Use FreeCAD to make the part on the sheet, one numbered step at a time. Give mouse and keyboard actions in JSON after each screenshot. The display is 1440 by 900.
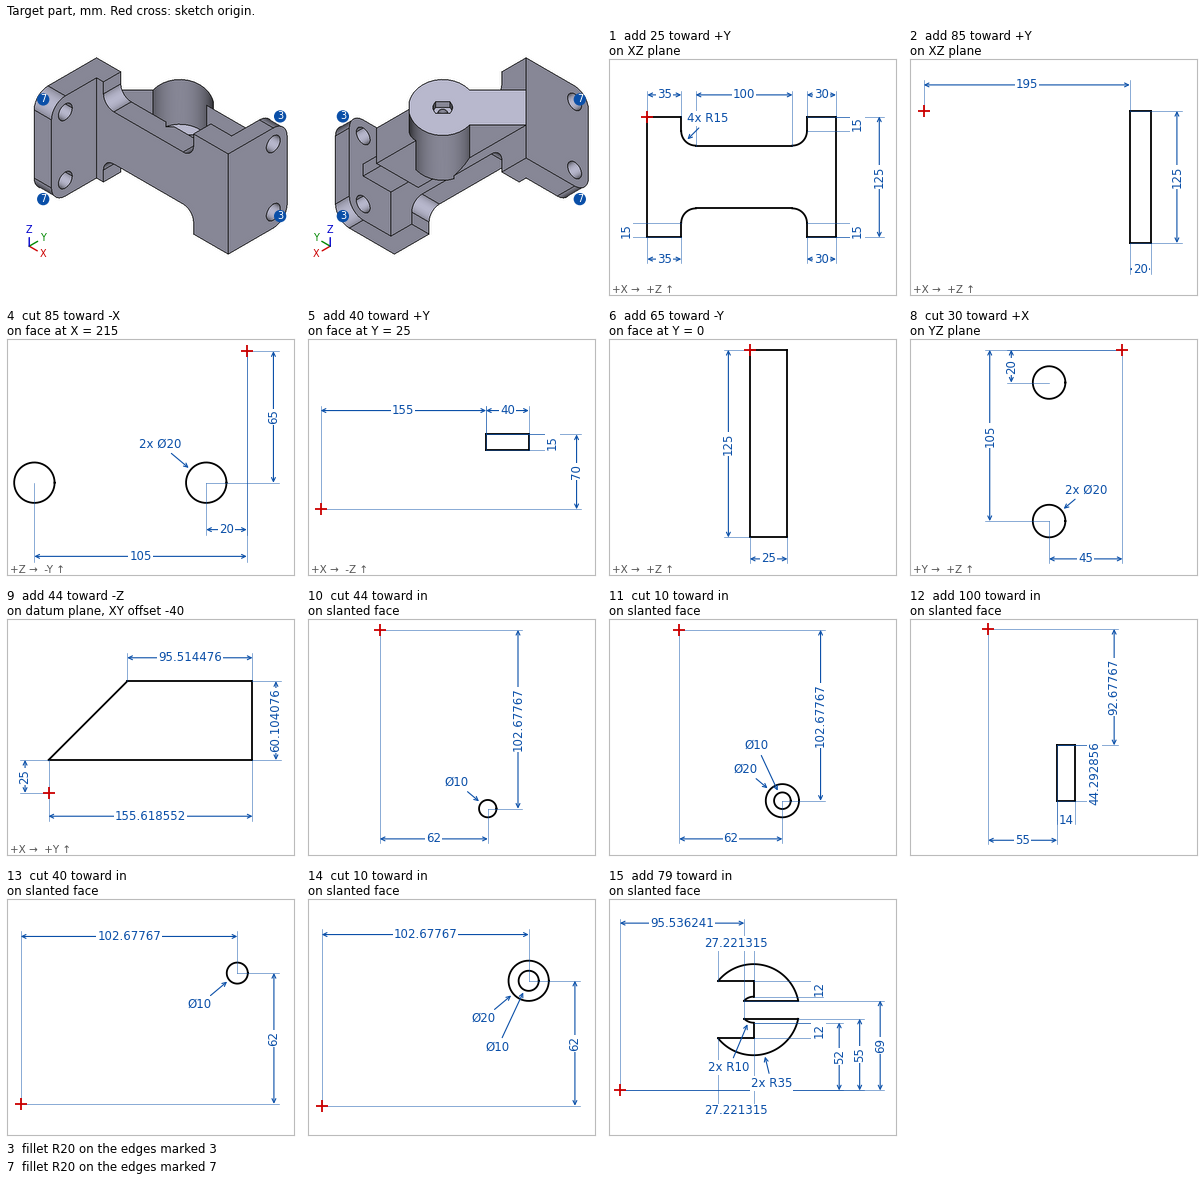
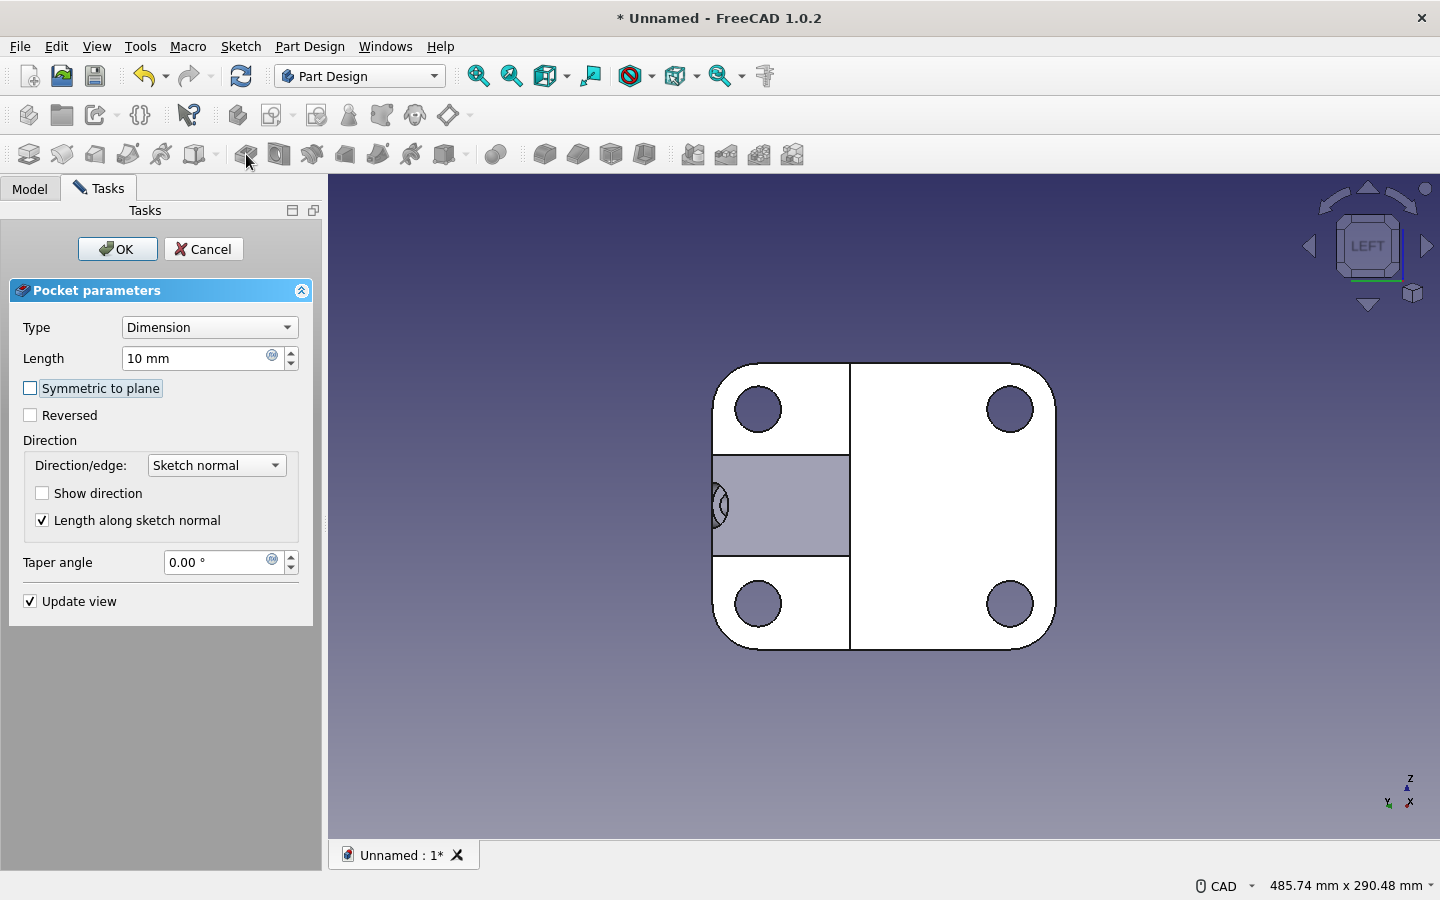
{"action": "left_click", "coordinate": [118, 249]}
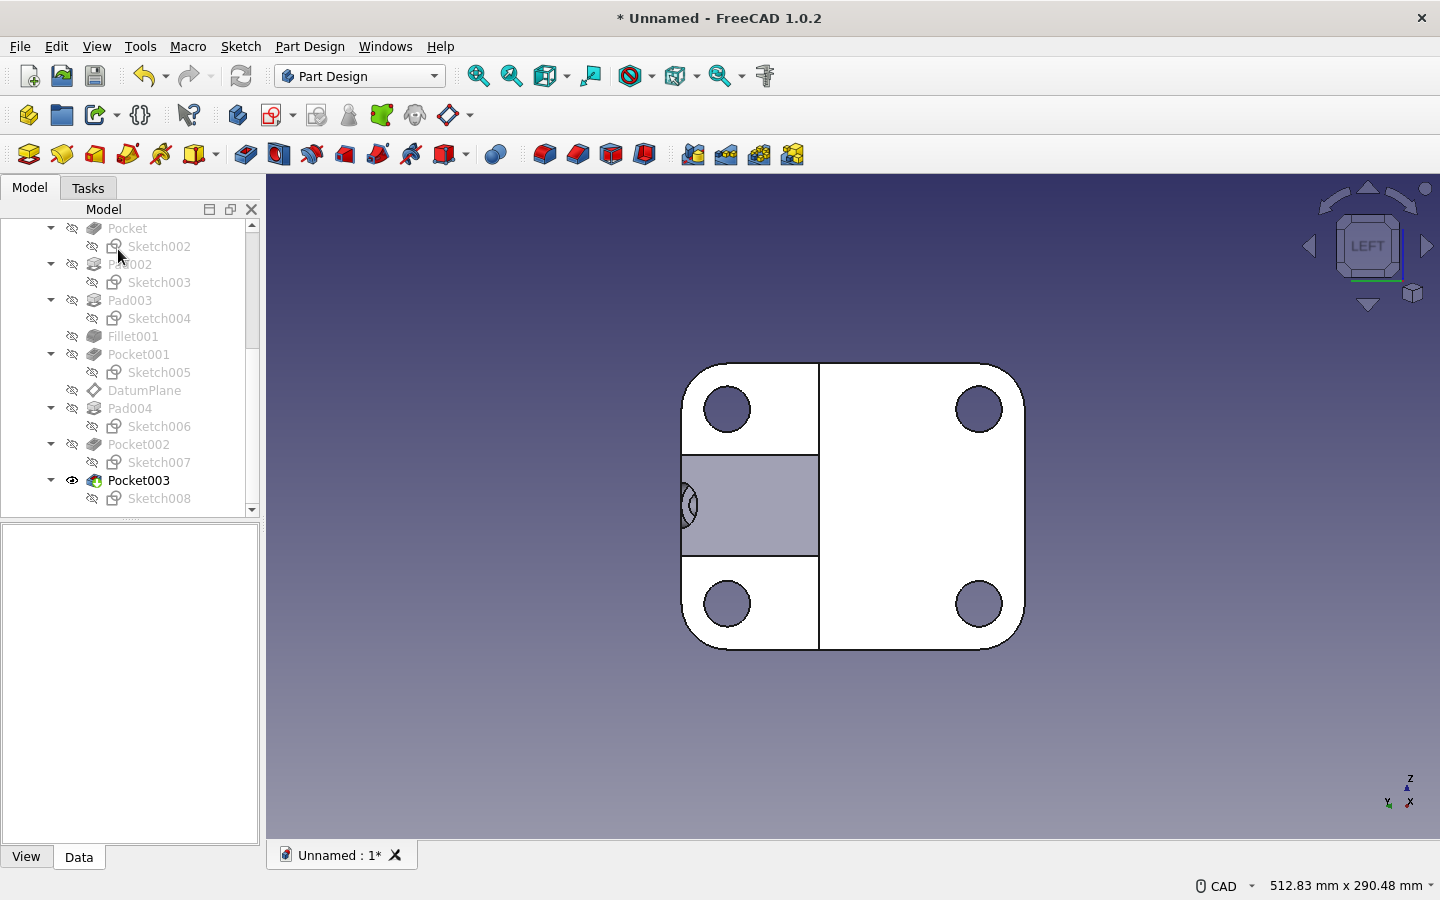
{"action": "key", "text": "v f"}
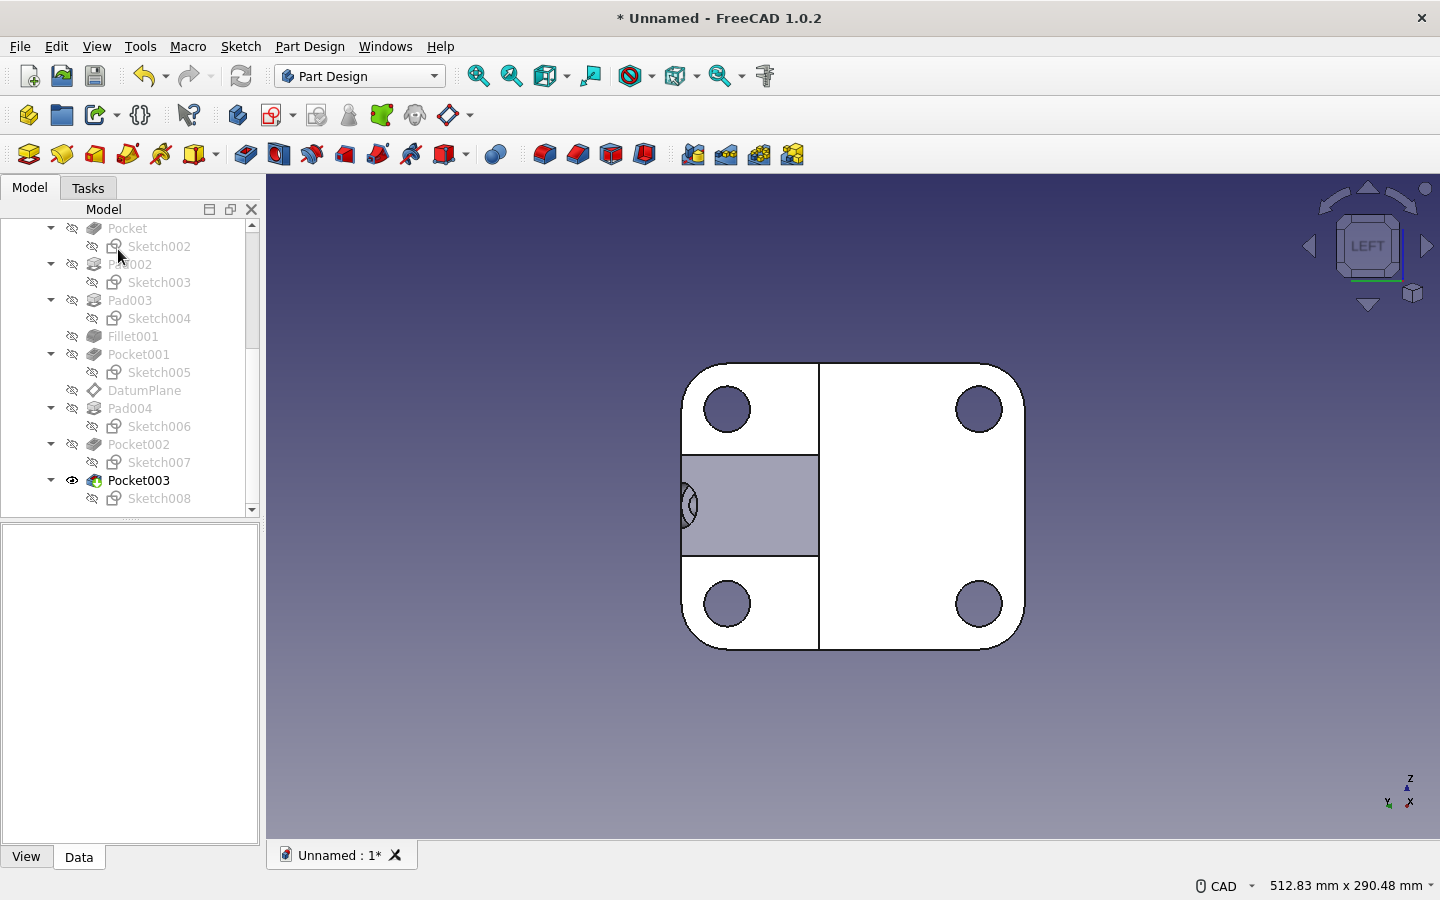
{"action": "left_click", "coordinate": [750, 504]}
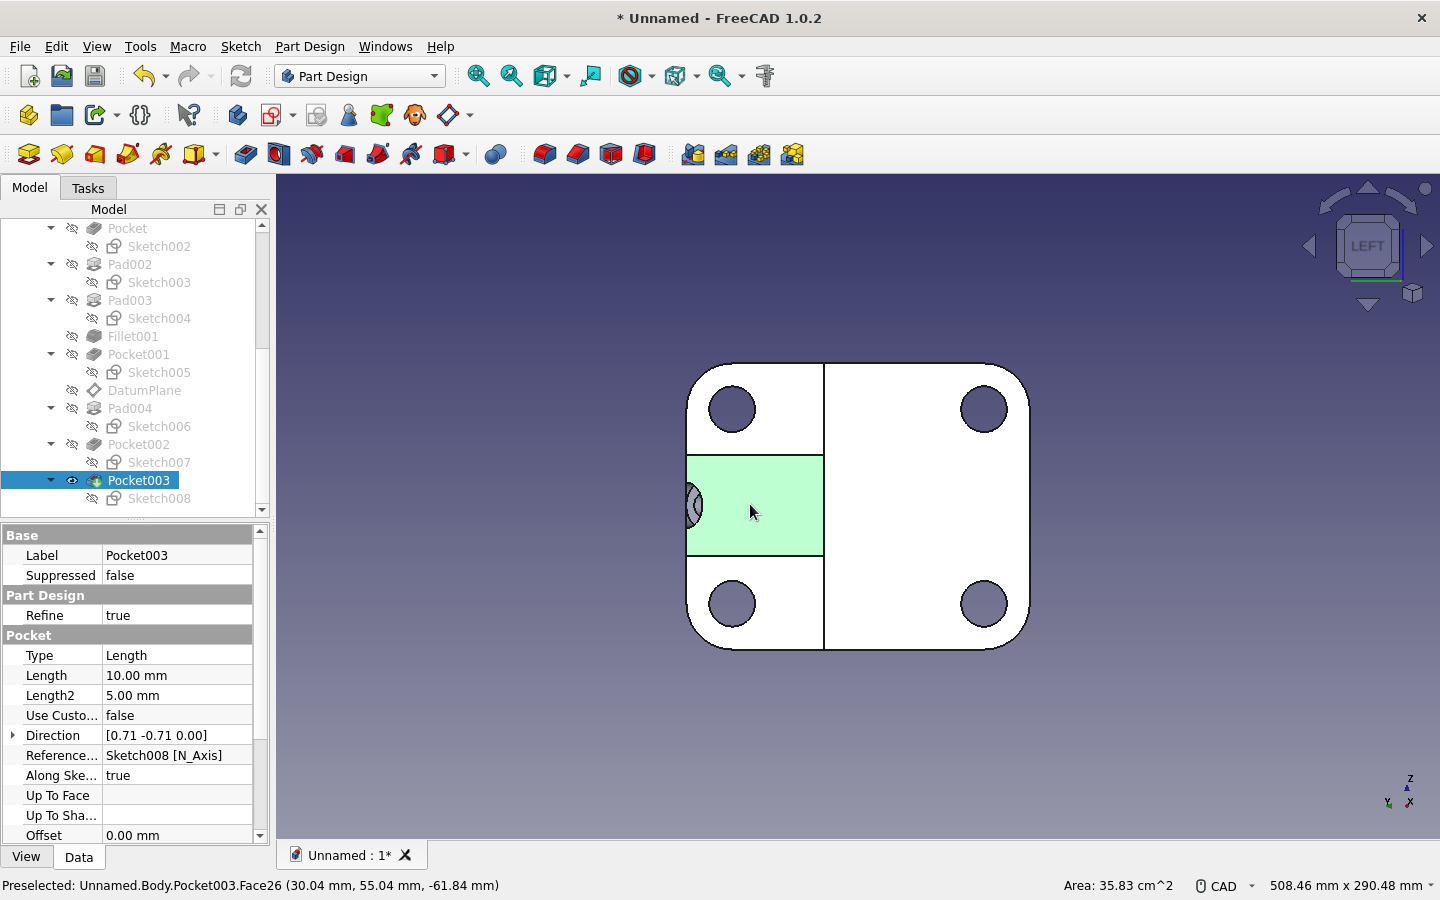
{"action": "left_click", "coordinate": [270, 116]}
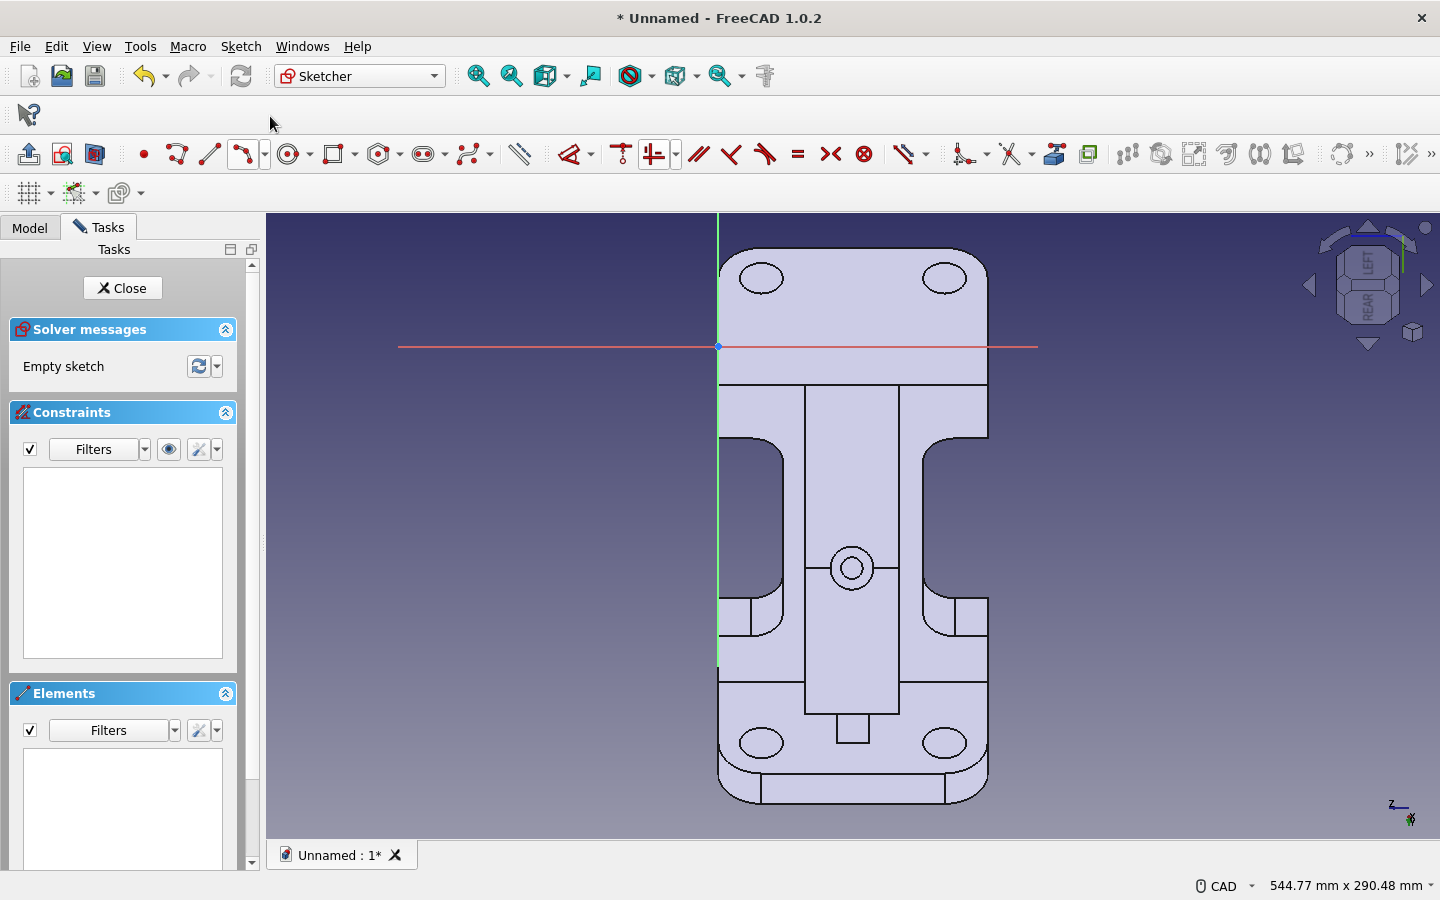
{"action": "scroll", "coordinate": [874, 617], "scroll_direction": "up", "scroll_amount": 7}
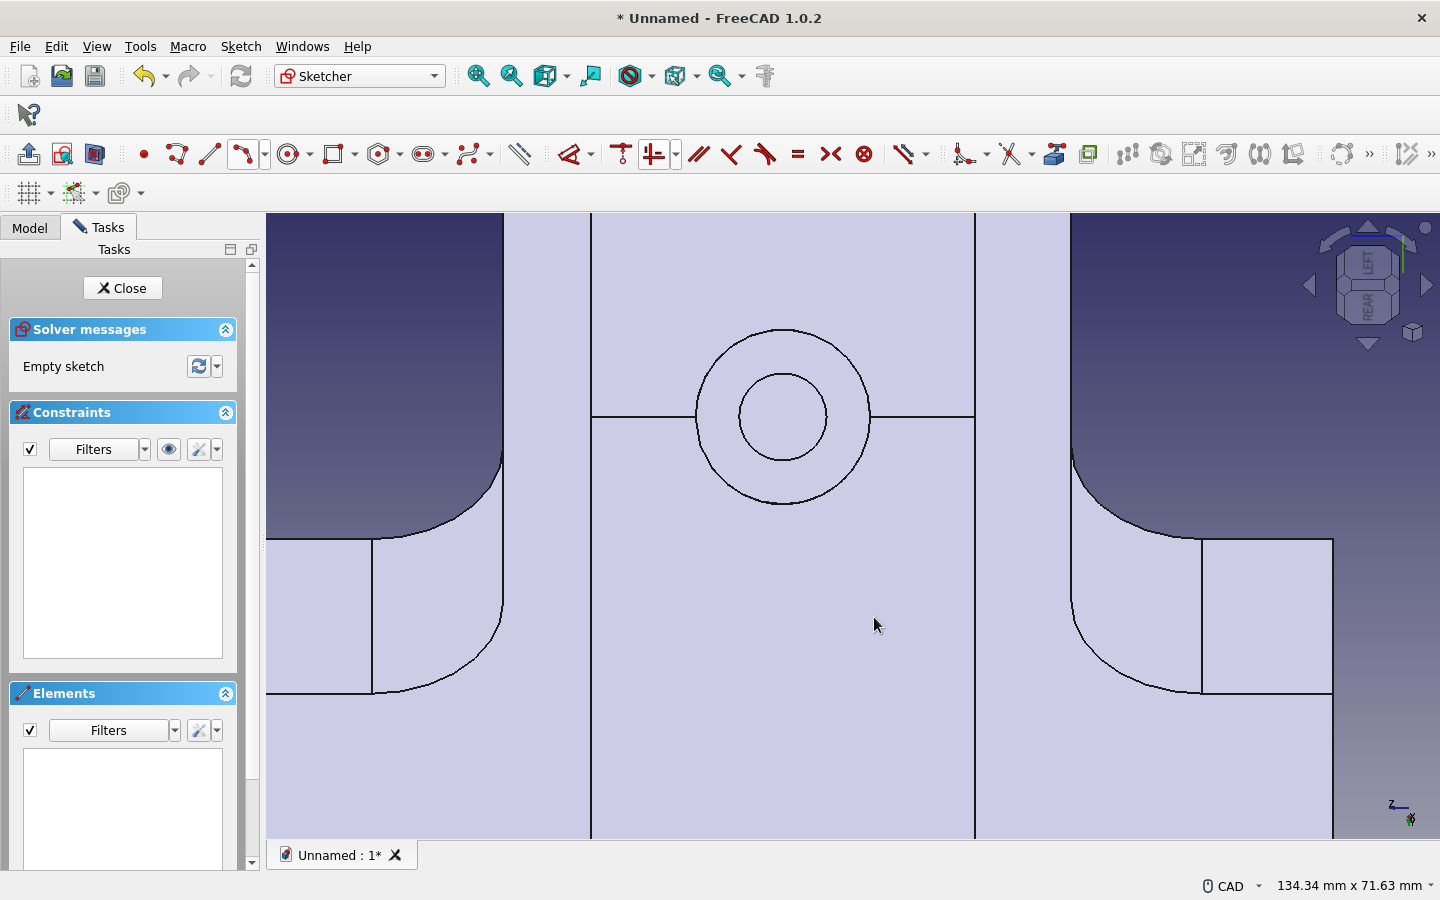
{"action": "key", "text": "g r"}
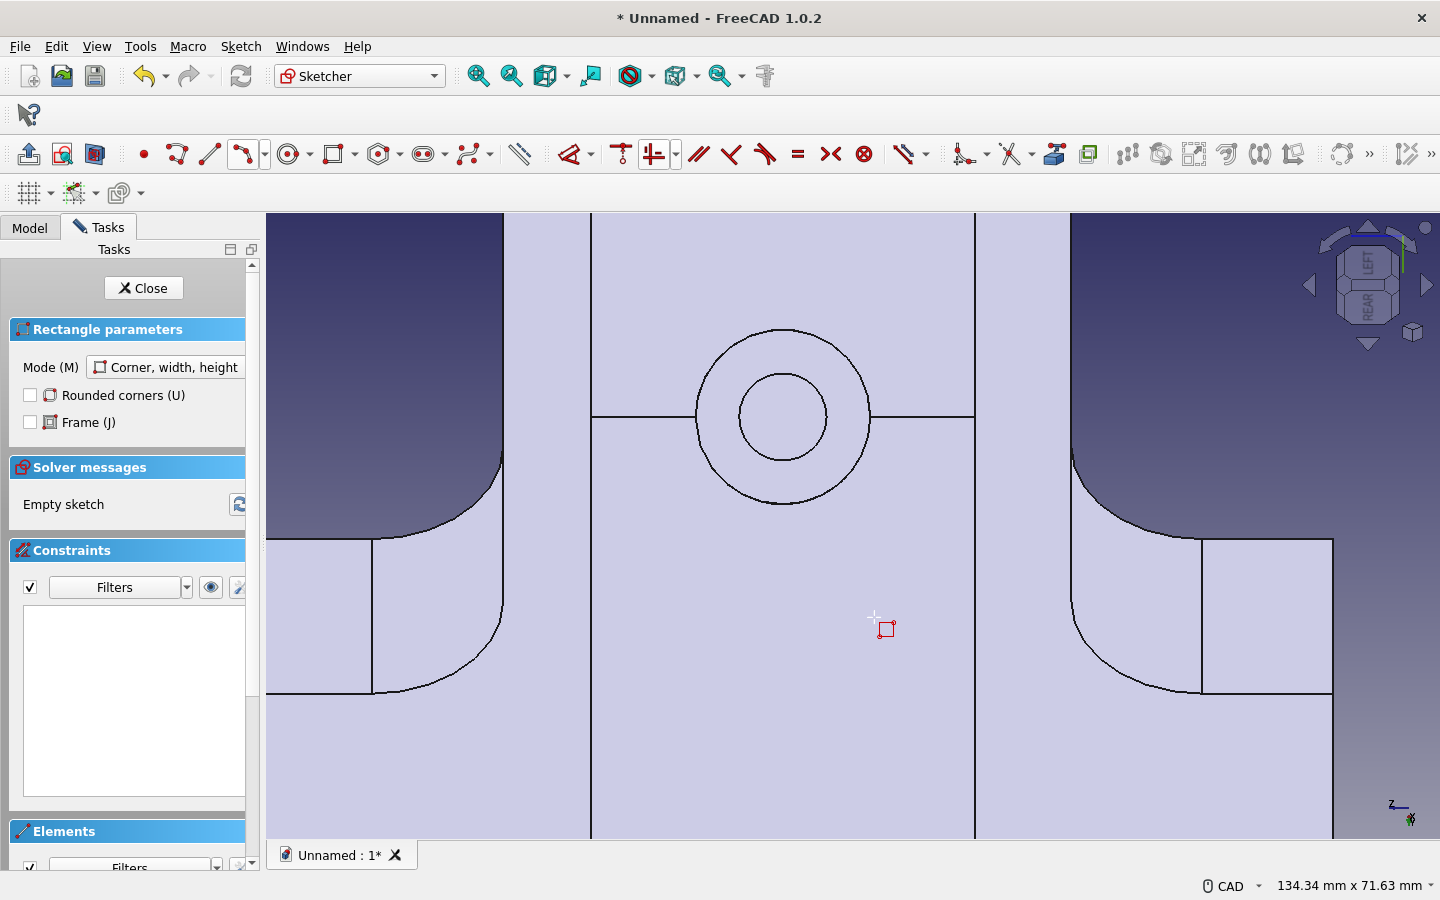
{"action": "left_click", "coordinate": [722, 330]}
{"action": "left_click", "coordinate": [844, 717]}
{"action": "key", "text": "Escape"}